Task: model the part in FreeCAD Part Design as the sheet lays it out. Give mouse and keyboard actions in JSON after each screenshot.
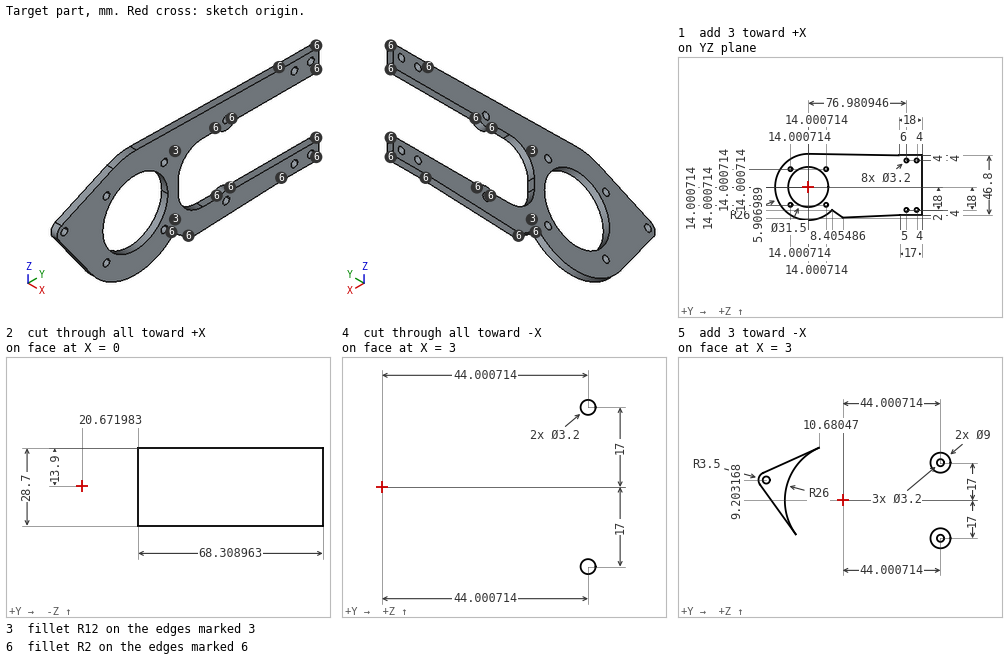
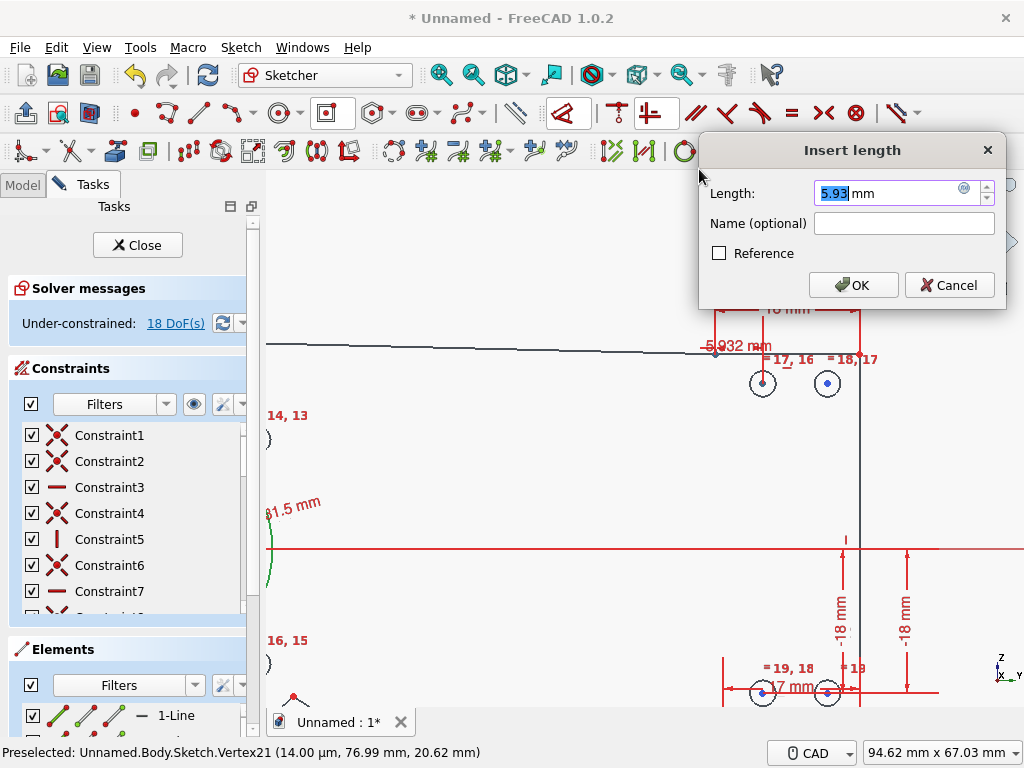
{"action": "type", "text": "6"}
{"action": "key", "text": "Return"}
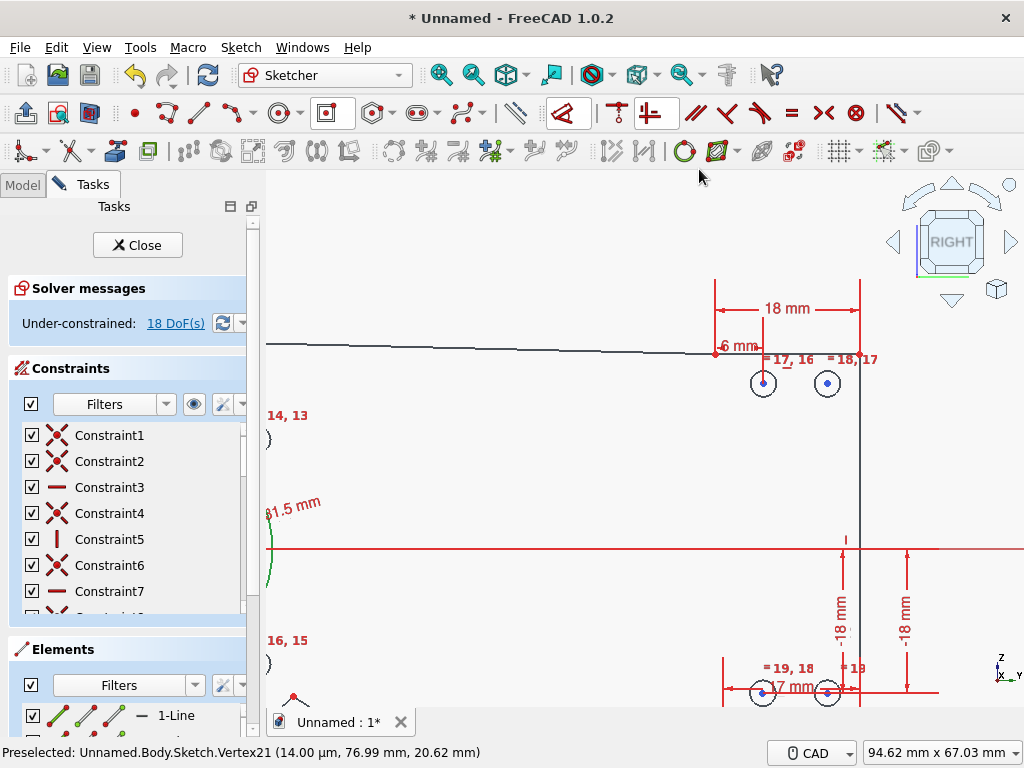
{"action": "scroll", "coordinate": [715, 354], "scroll_direction": "up", "scroll_amount": 2}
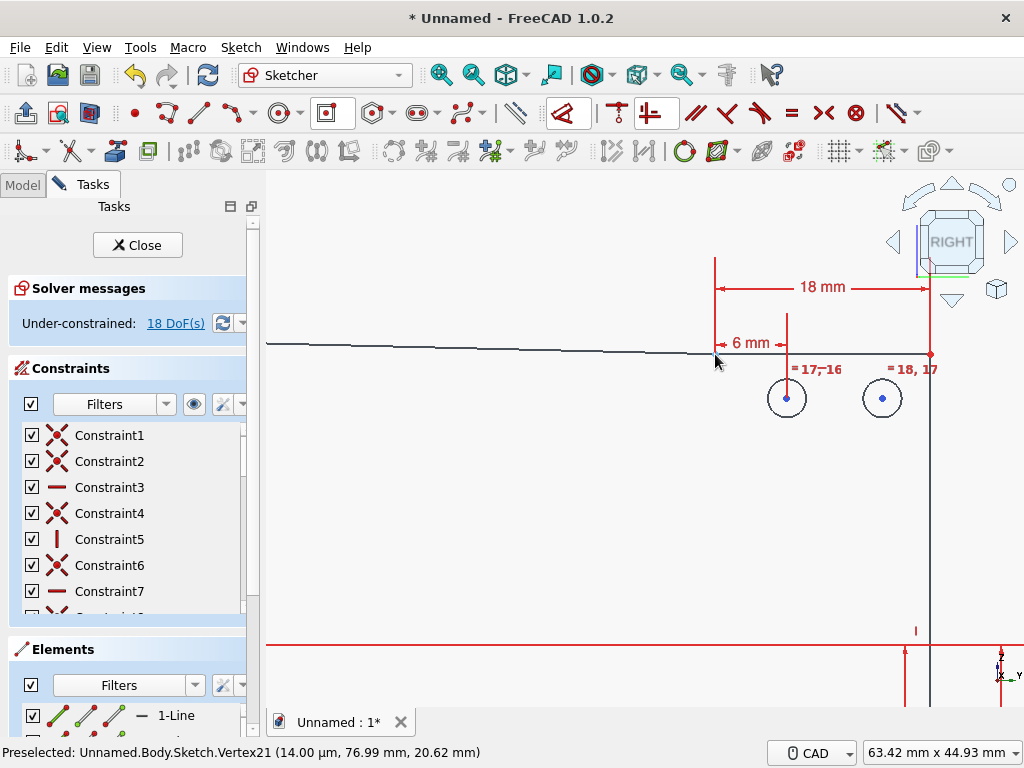
{"action": "left_click", "coordinate": [715, 354]}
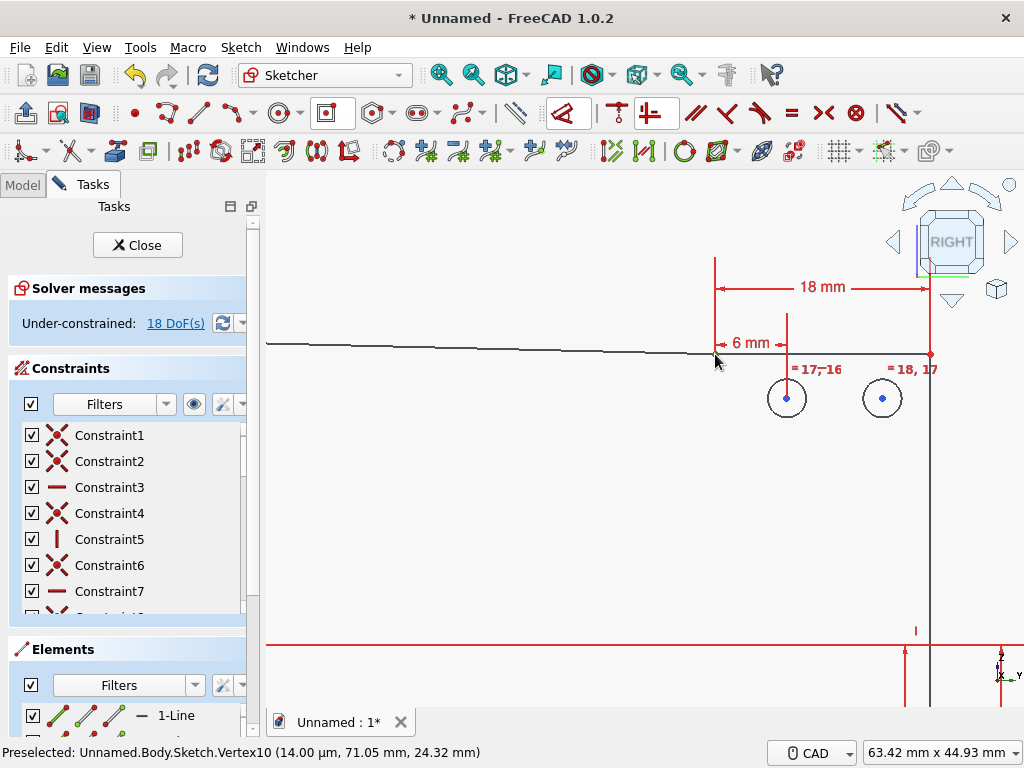
{"action": "left_click", "coordinate": [787, 398]}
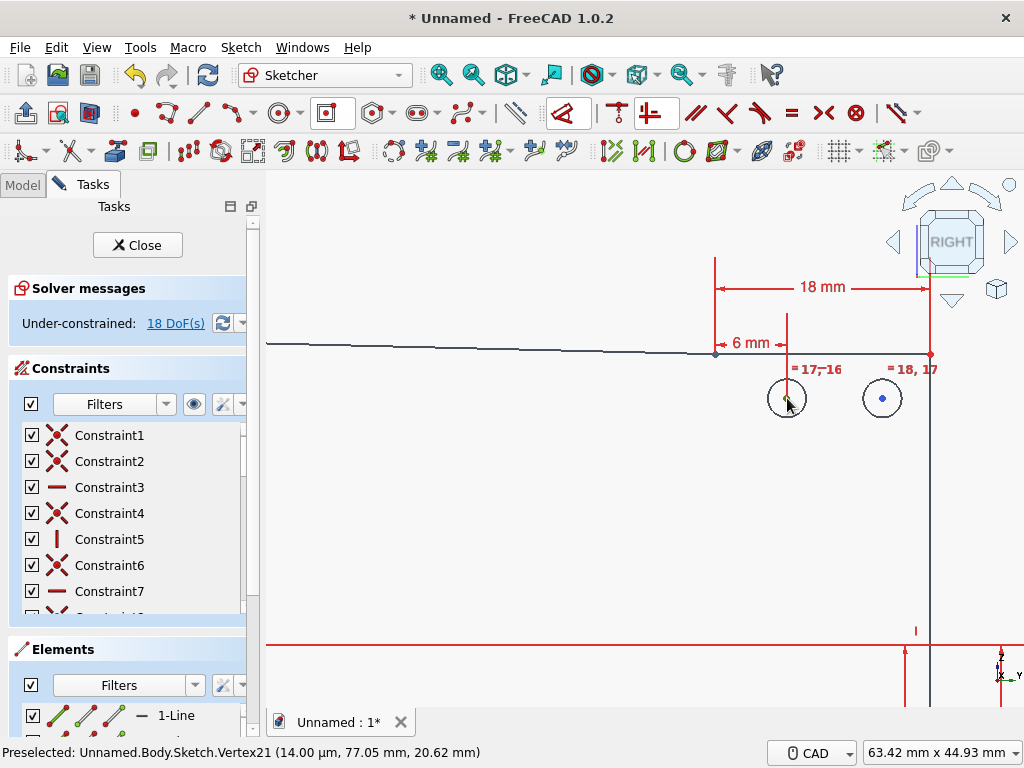
{"action": "left_click", "coordinate": [586, 114]}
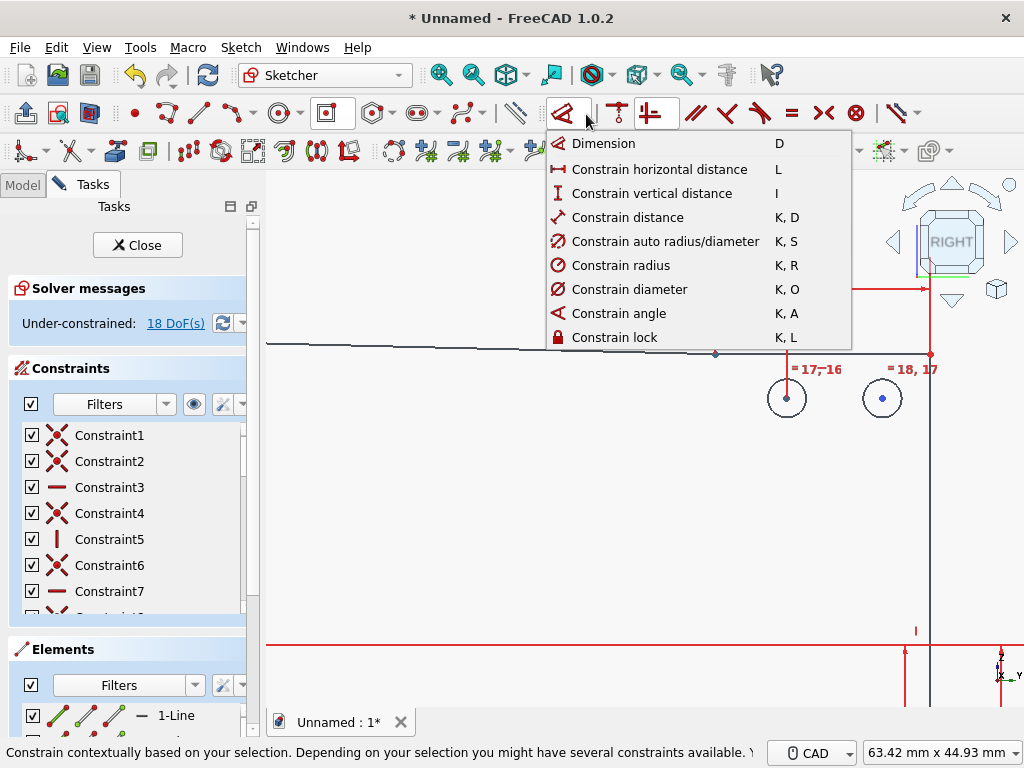
{"action": "left_click", "coordinate": [699, 193]}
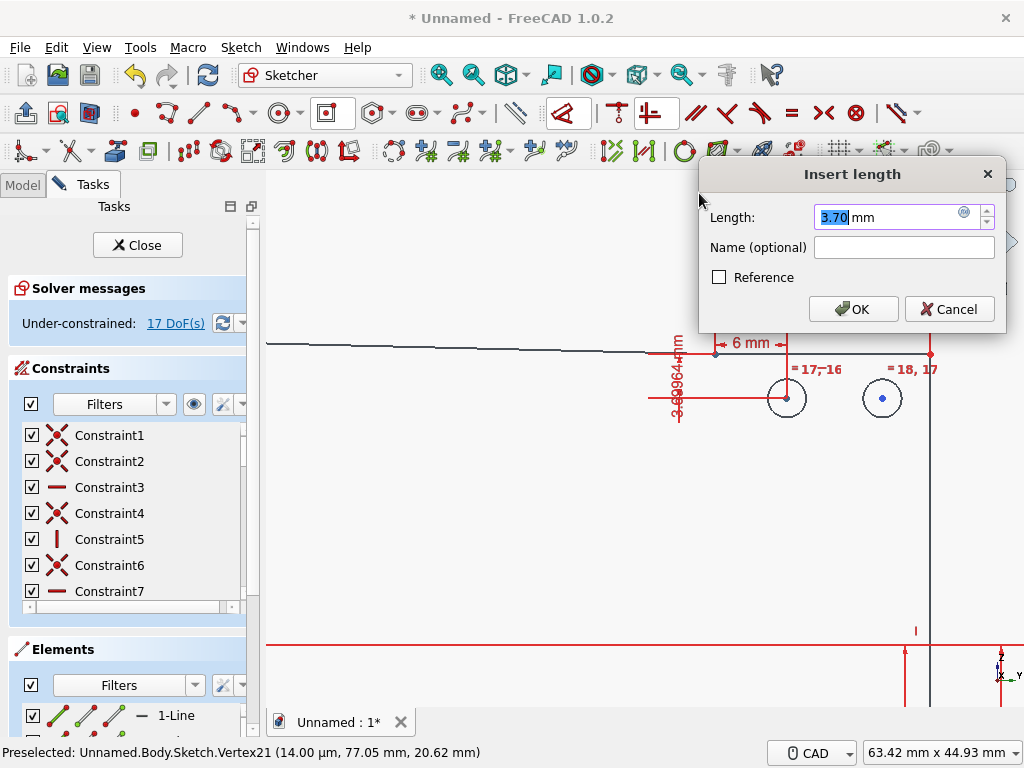
{"action": "type", "text": "4"}
{"action": "key", "text": "Return"}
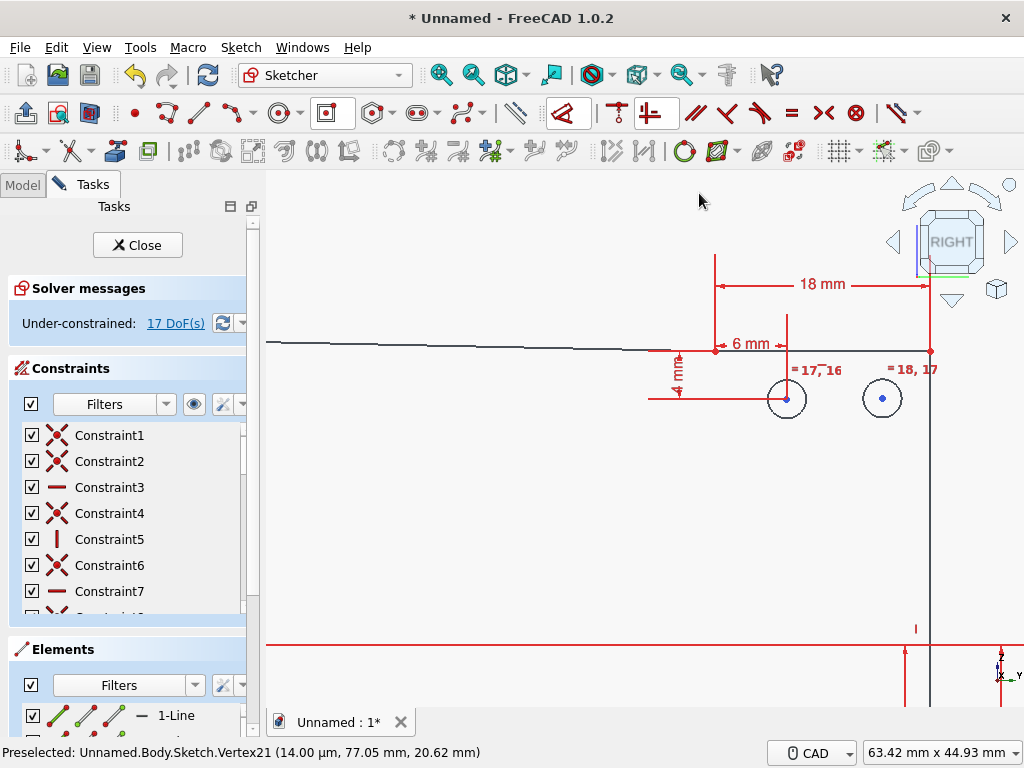
{"action": "scroll", "coordinate": [715, 355], "scroll_direction": "down", "scroll_amount": 6}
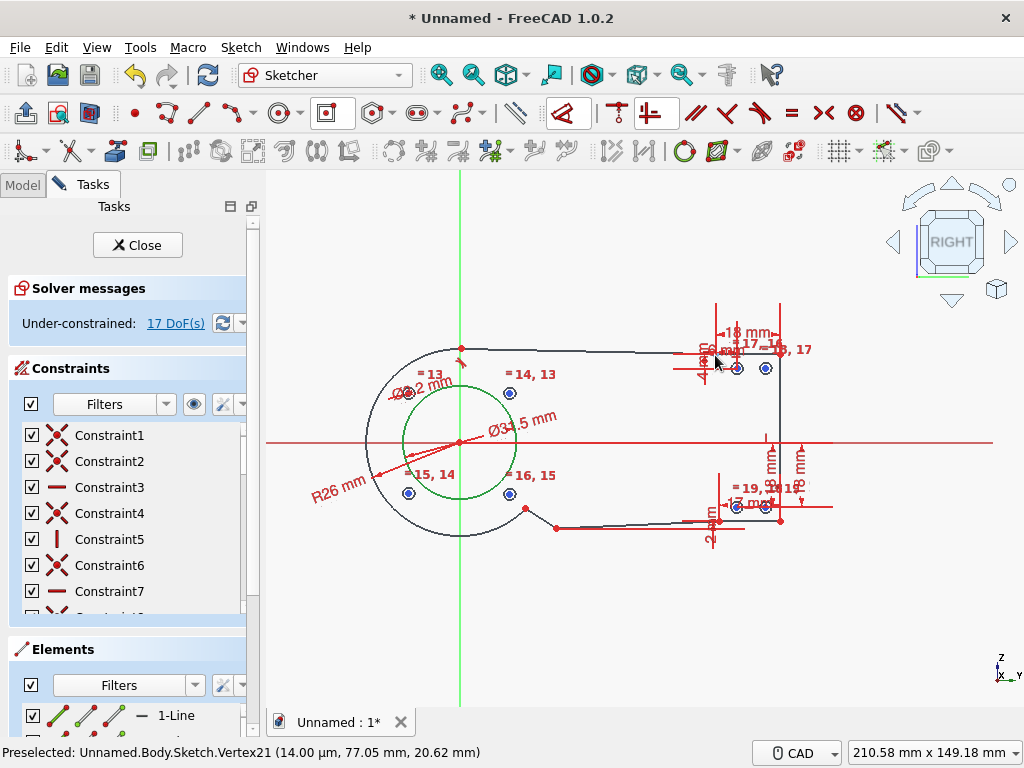
{"action": "scroll", "coordinate": [780, 354], "scroll_direction": "up", "scroll_amount": 6}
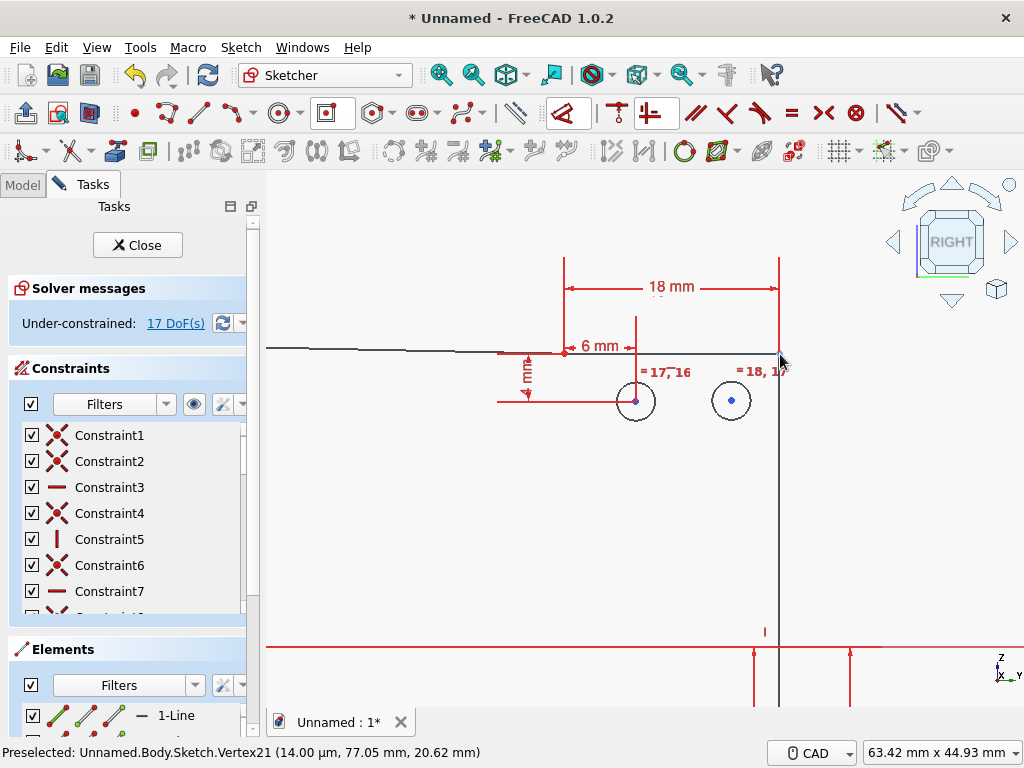
{"action": "left_click", "coordinate": [779, 354]}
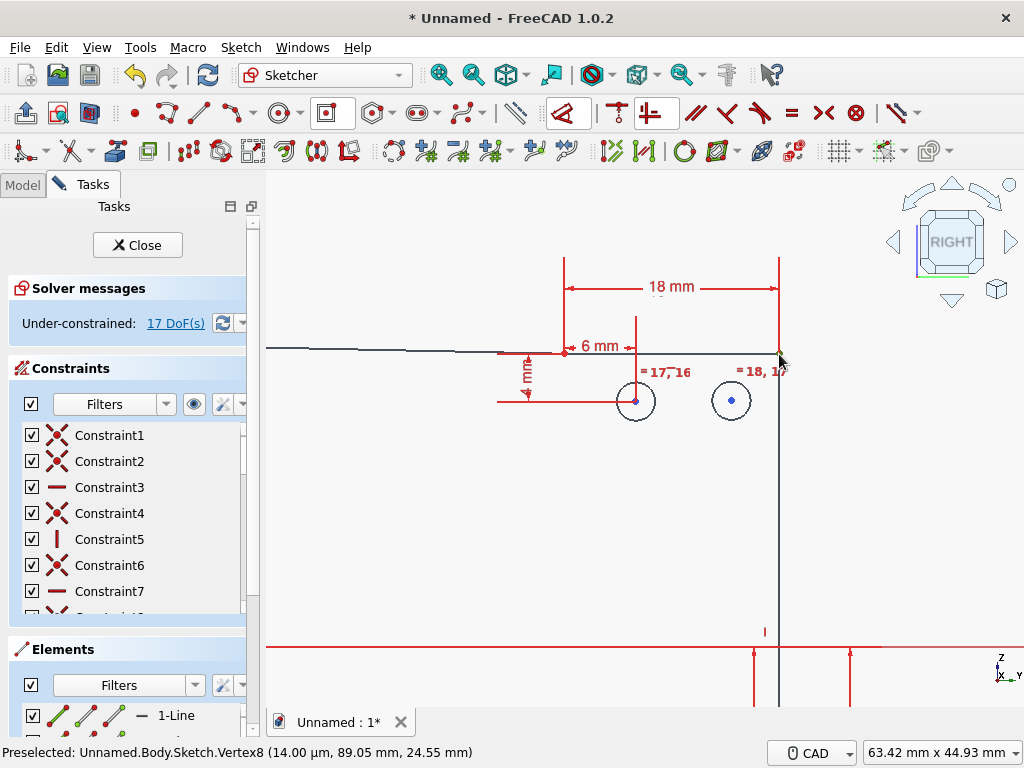
{"action": "left_click", "coordinate": [731, 401]}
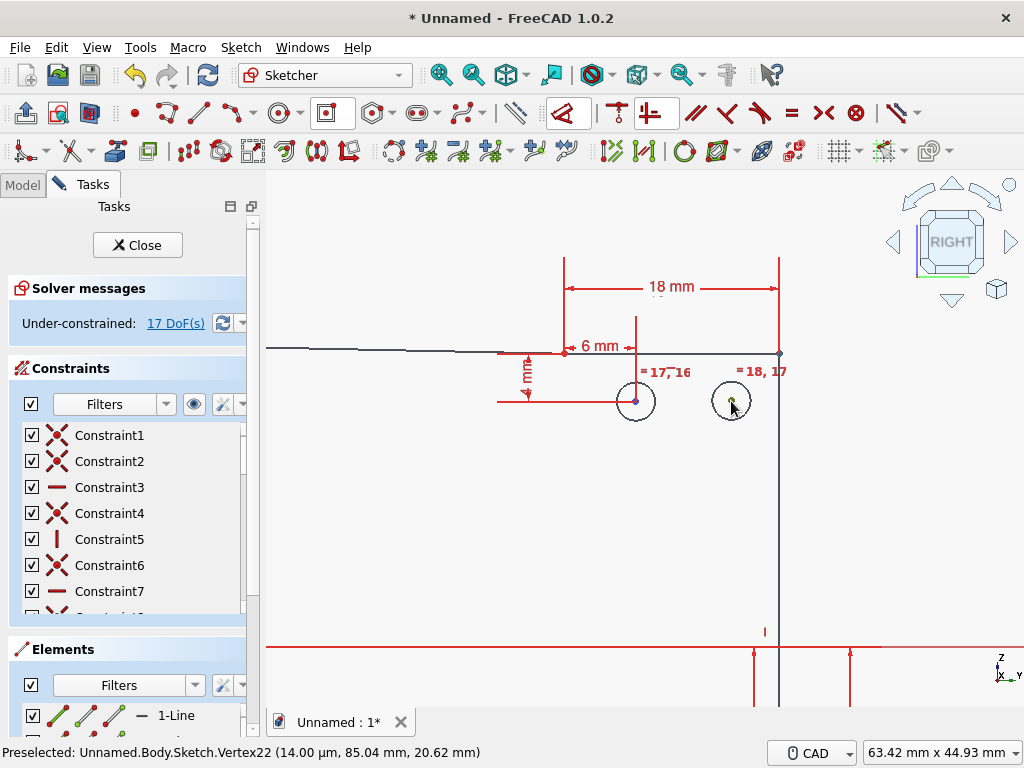
{"action": "left_click", "coordinate": [586, 114]}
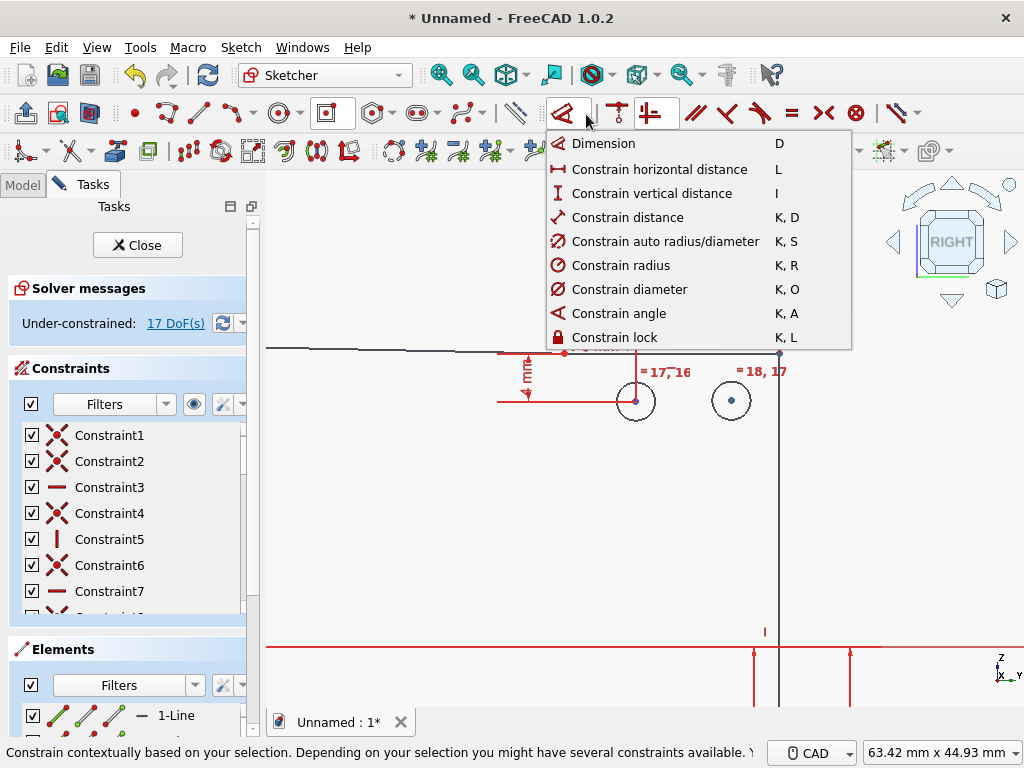
{"action": "left_click", "coordinate": [699, 169]}